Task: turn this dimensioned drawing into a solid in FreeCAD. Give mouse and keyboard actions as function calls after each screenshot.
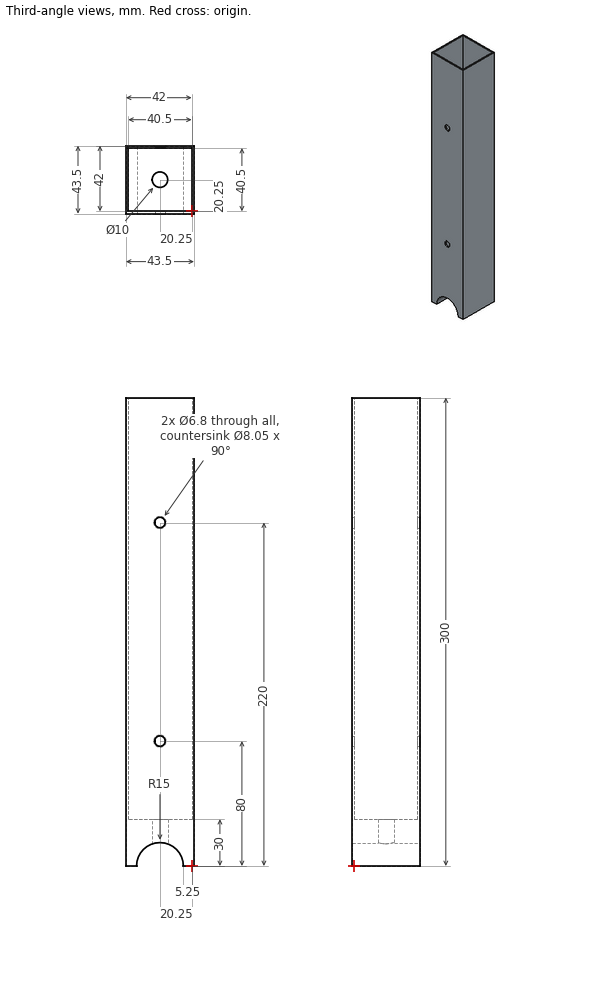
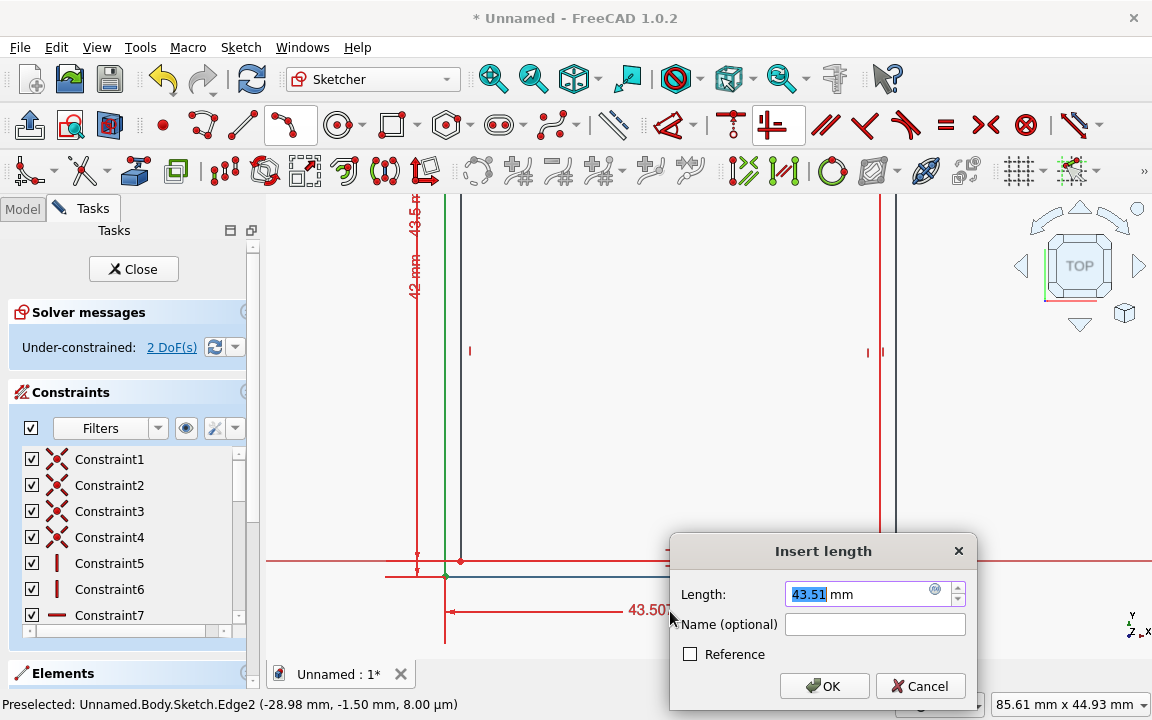
text(43.5)
key(Return)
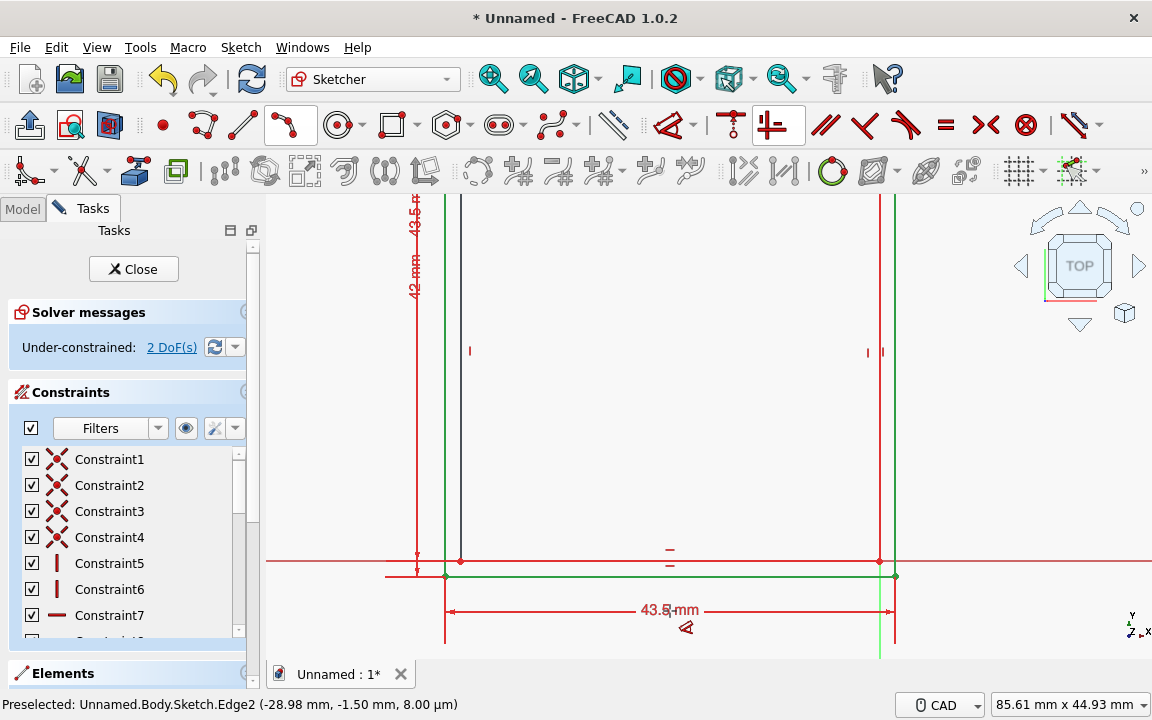
click(880, 436)
click(914, 392)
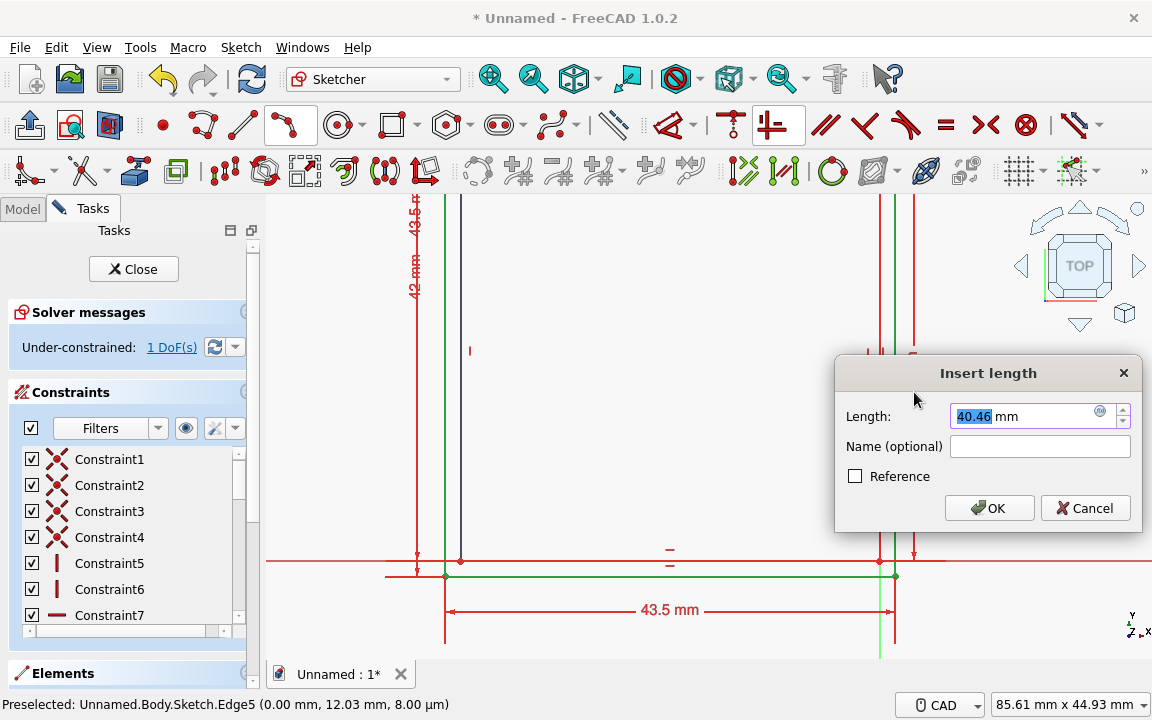
text(40.5)
key(Return)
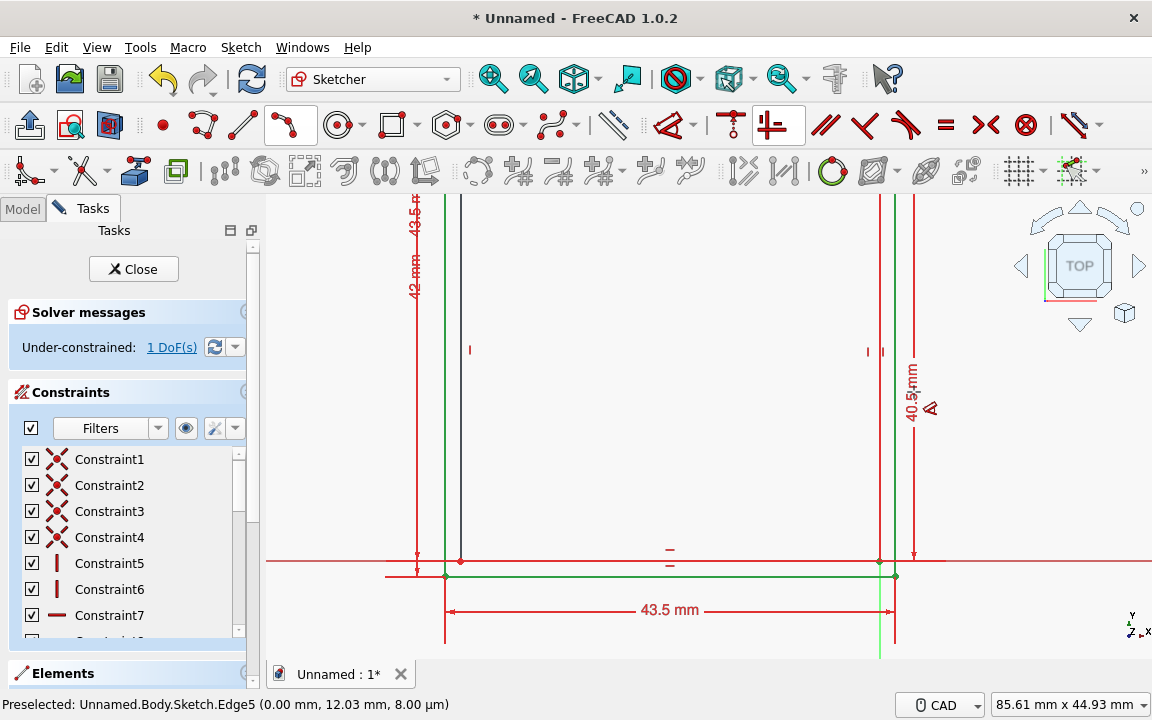
scroll(580, 578, down, 2)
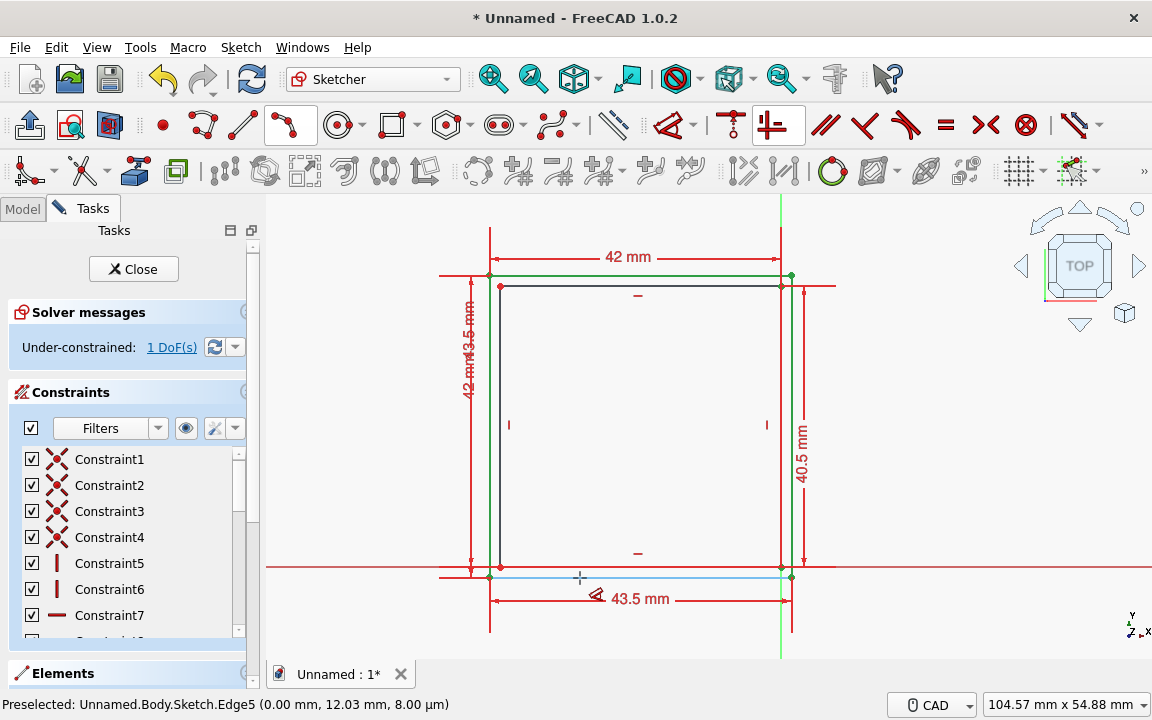
scroll(697, 286, up, 2)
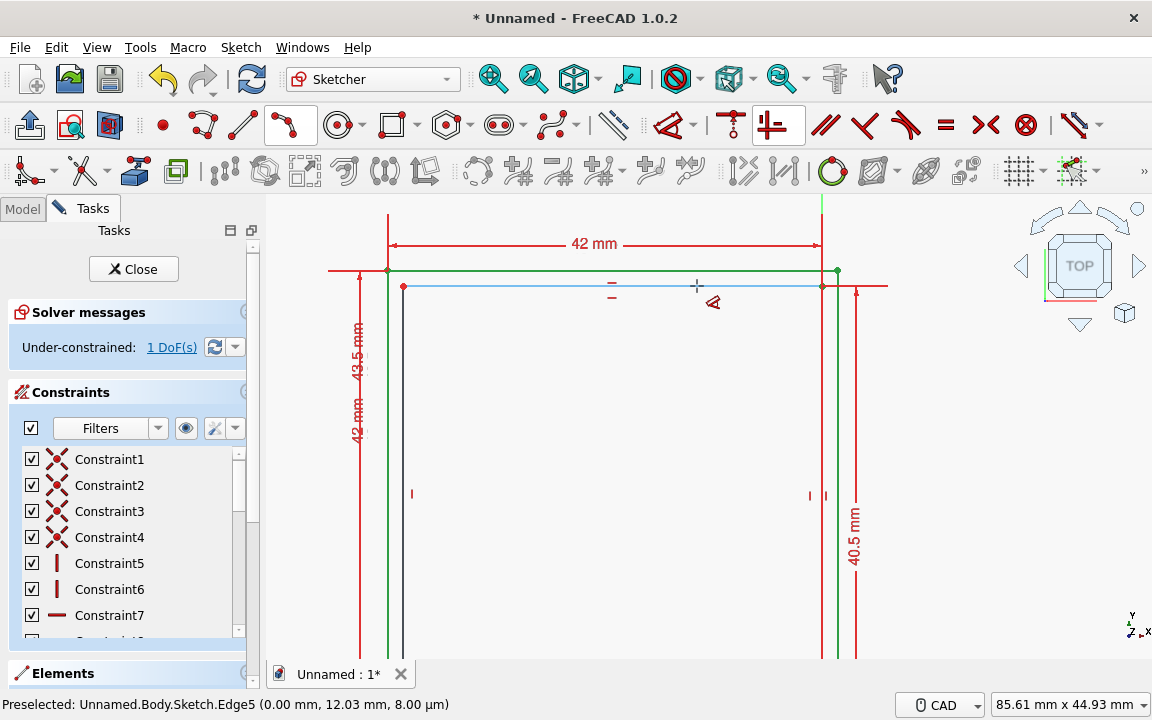
click(697, 286)
click(516, 252)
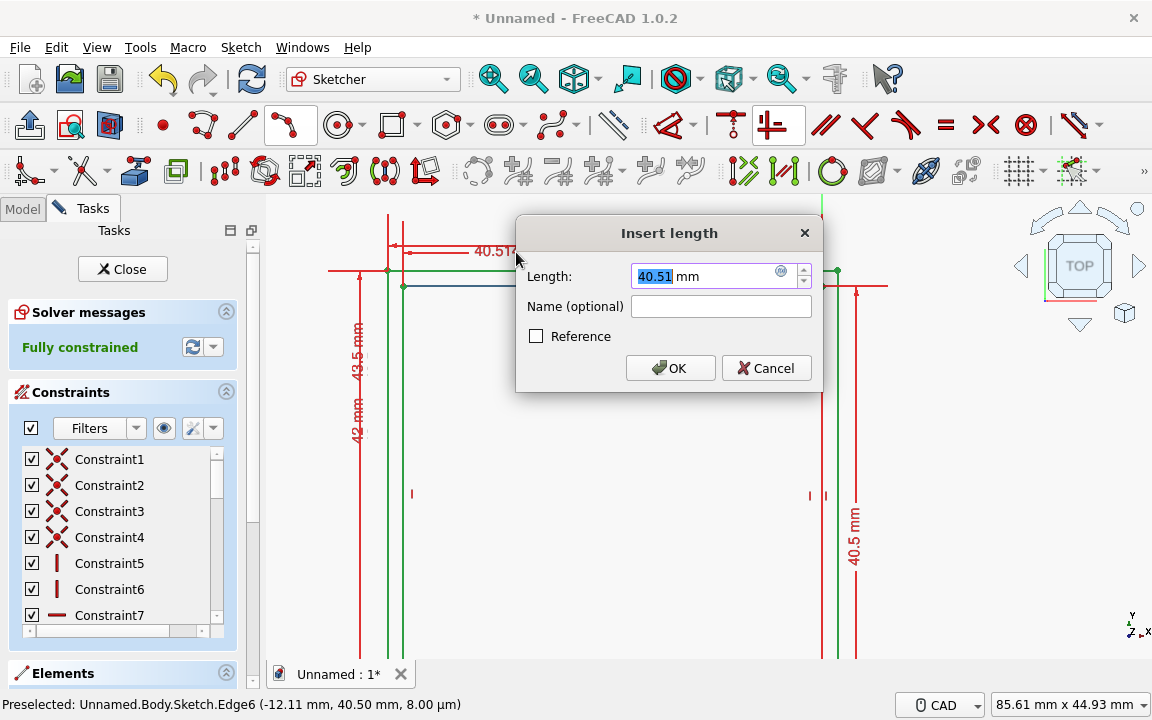
text(40.5)
key(Return)
key(Escape)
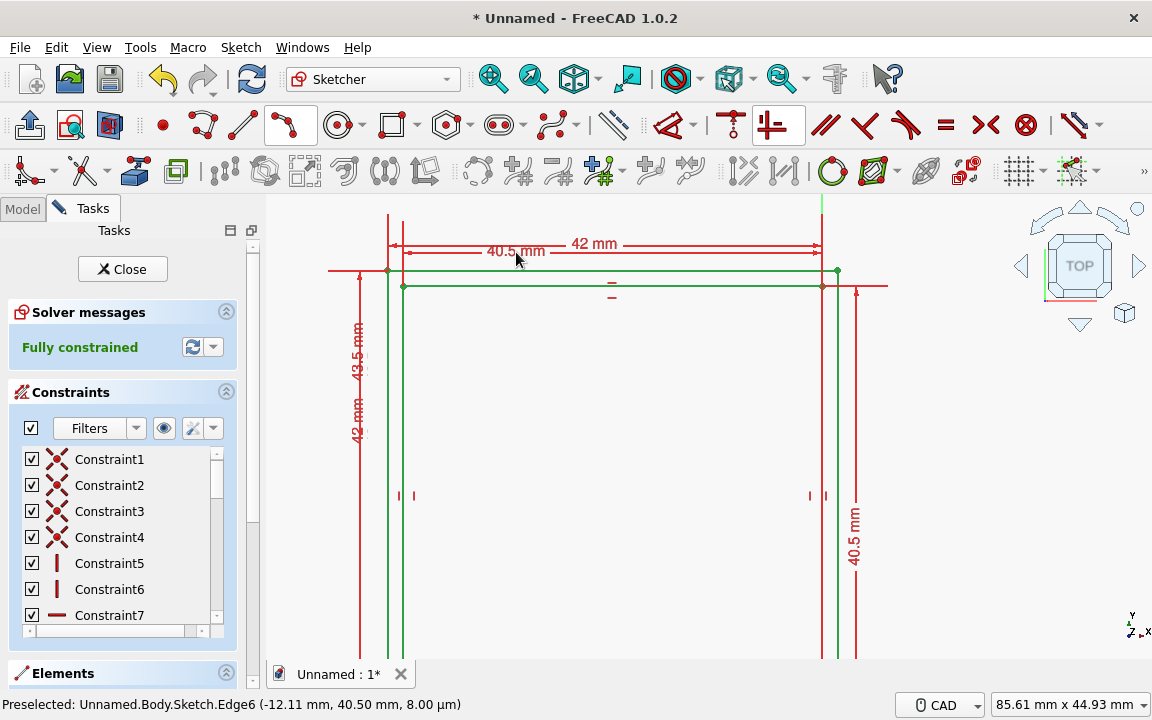
click(123, 269)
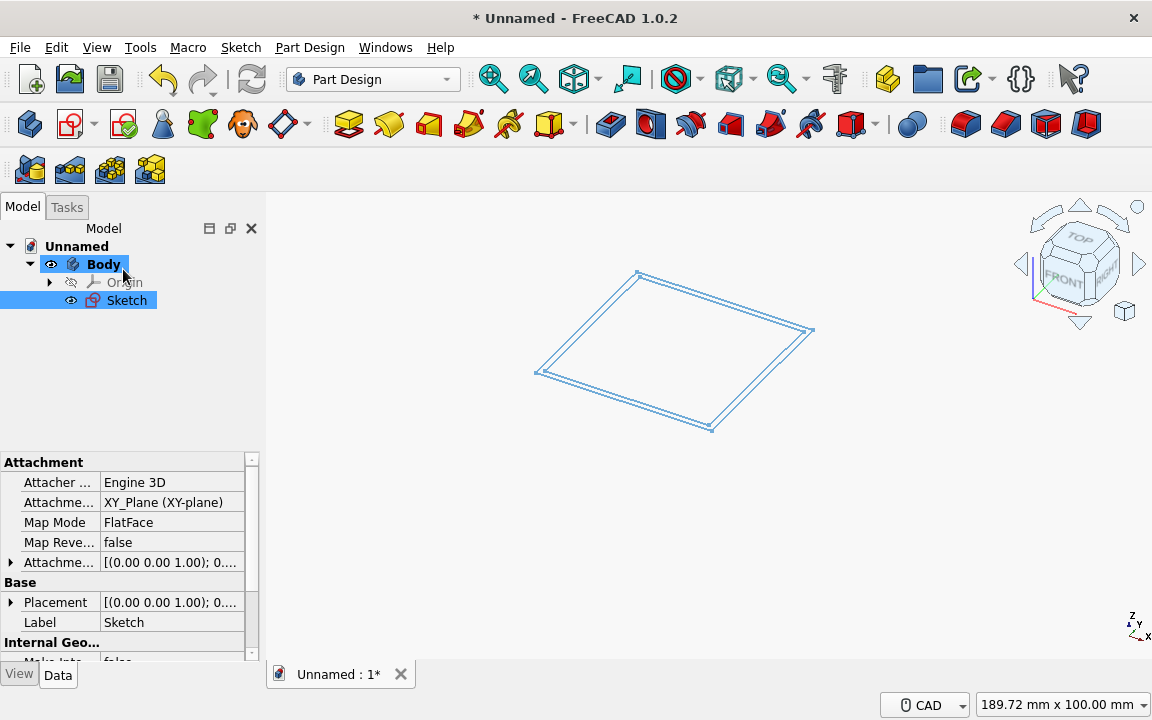
click(350, 124)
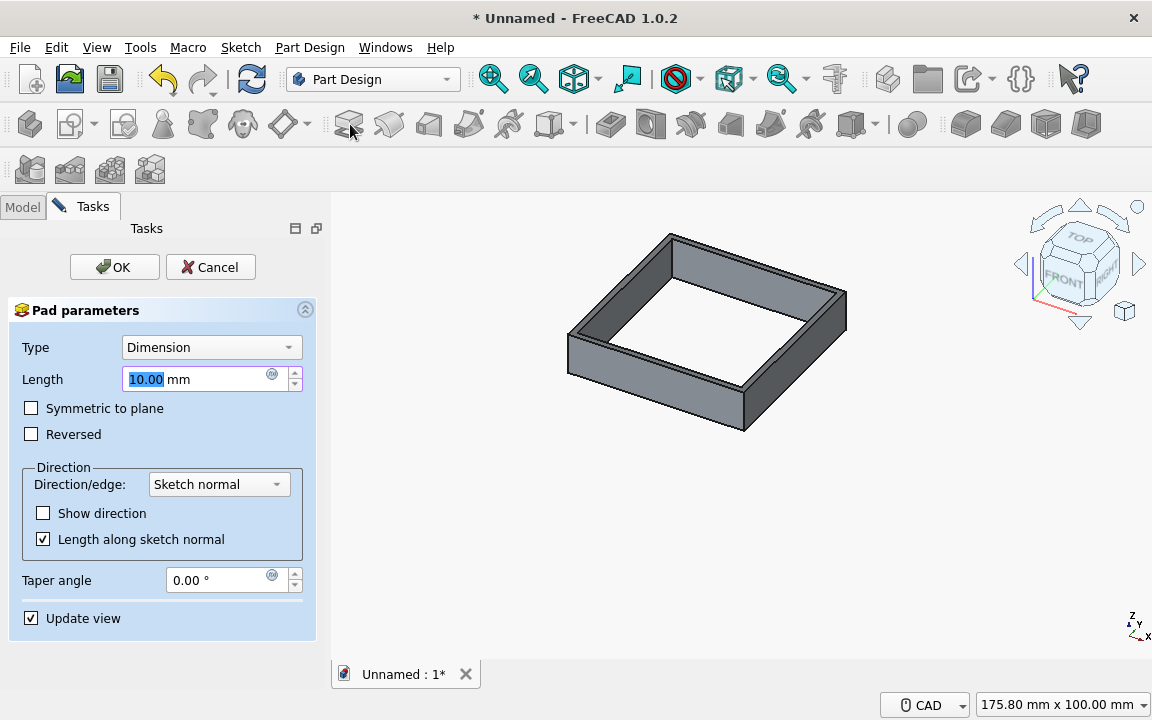
text(300)
key(Tab)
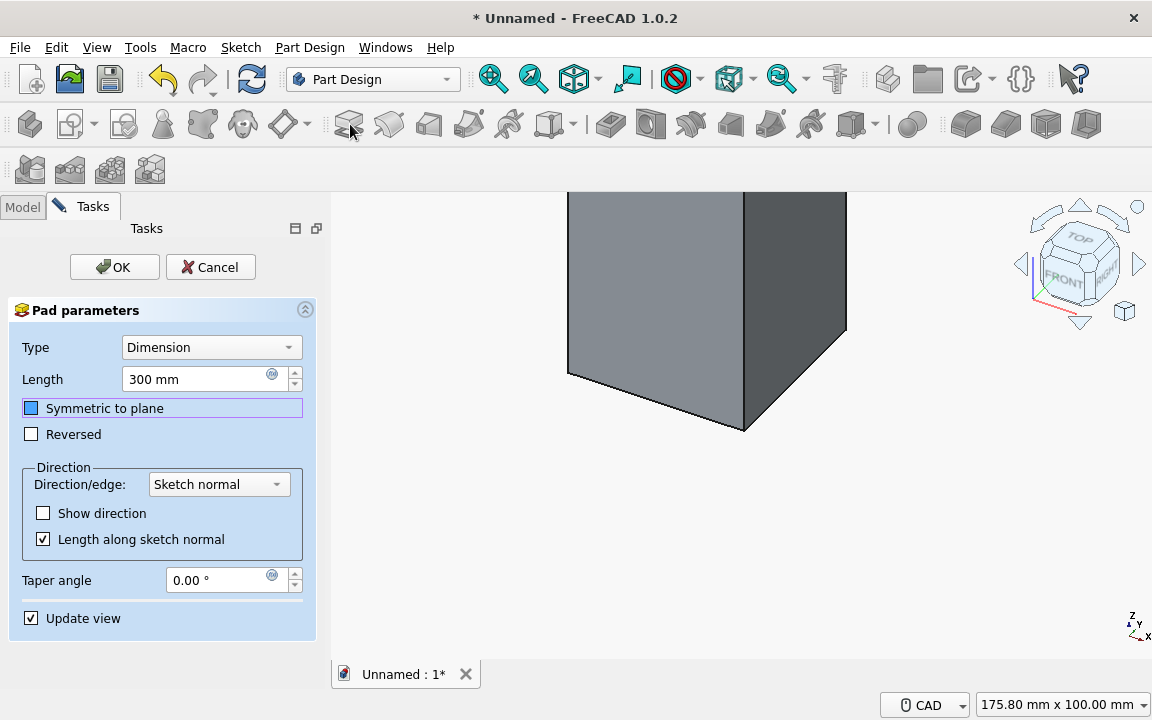
click(115, 267)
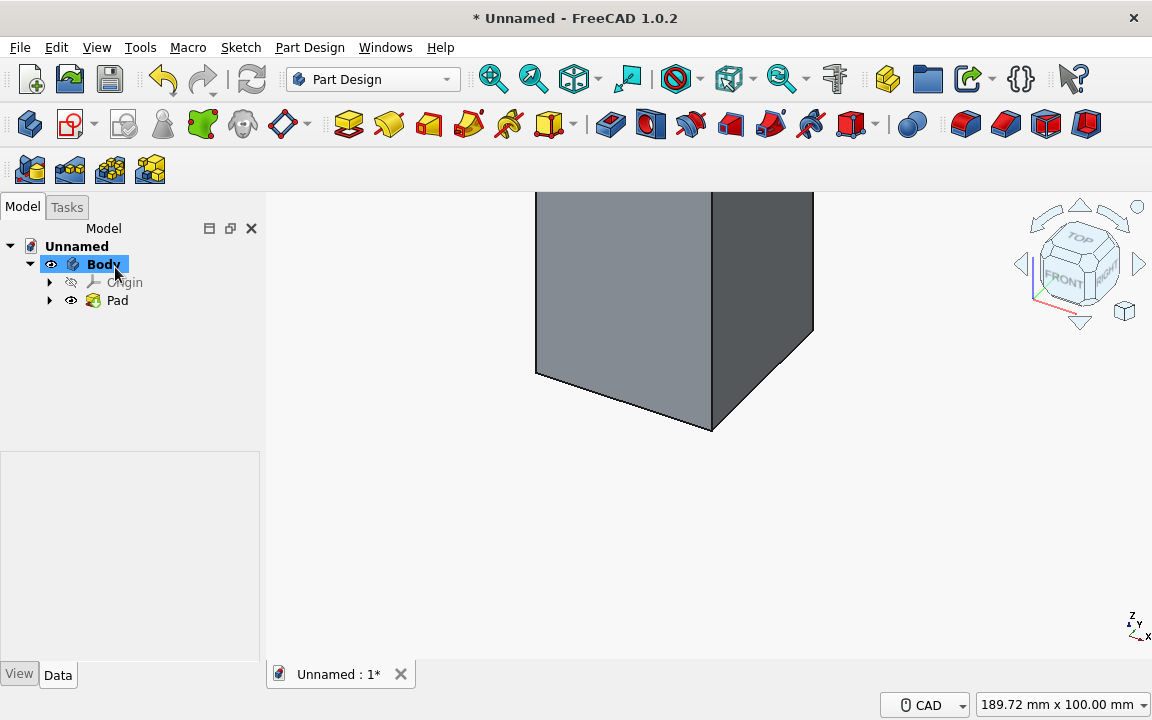
click(494, 80)